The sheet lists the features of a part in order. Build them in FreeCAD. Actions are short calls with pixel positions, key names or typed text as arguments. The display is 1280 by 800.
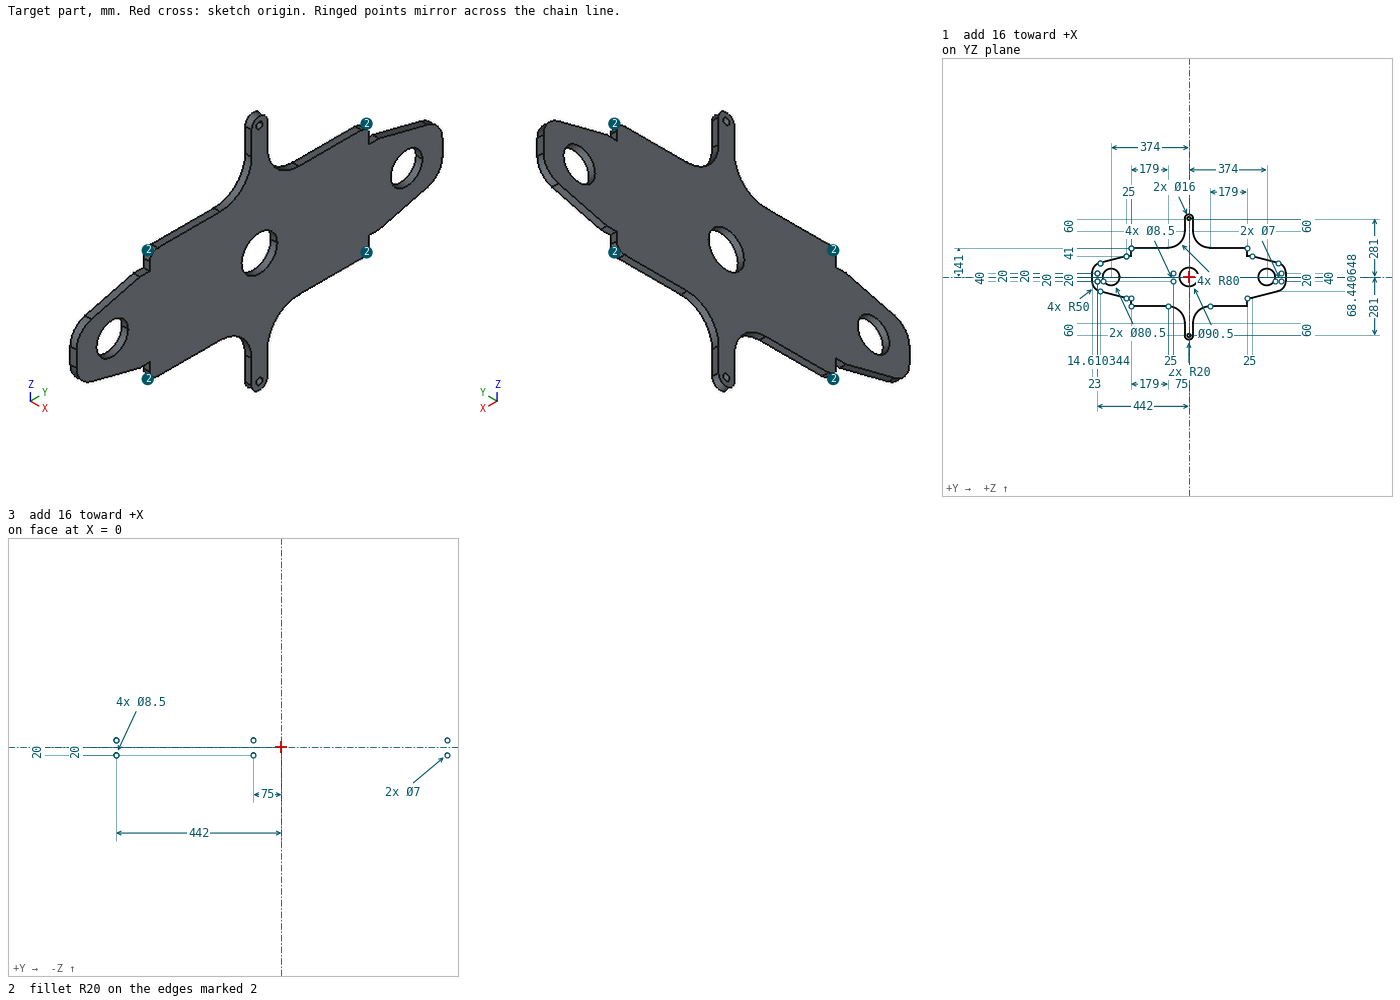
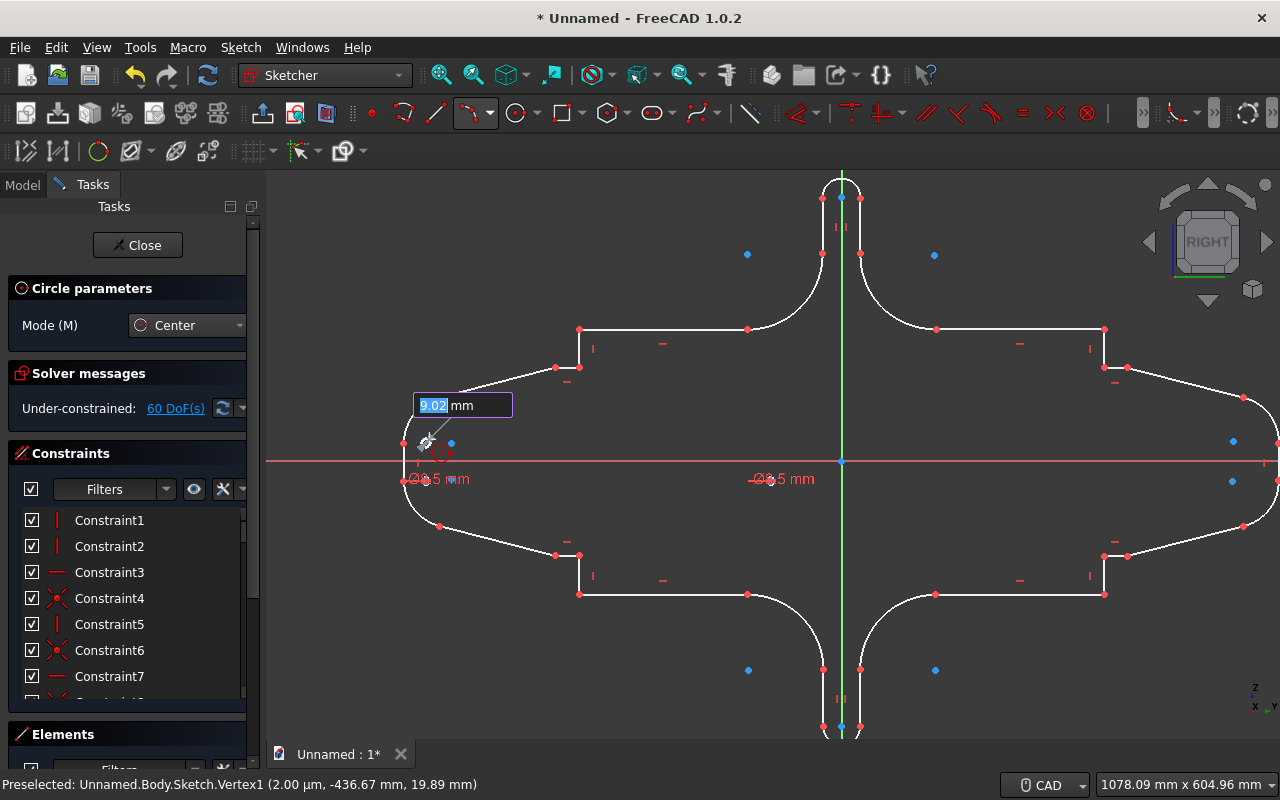
text(8.5)
key(Return)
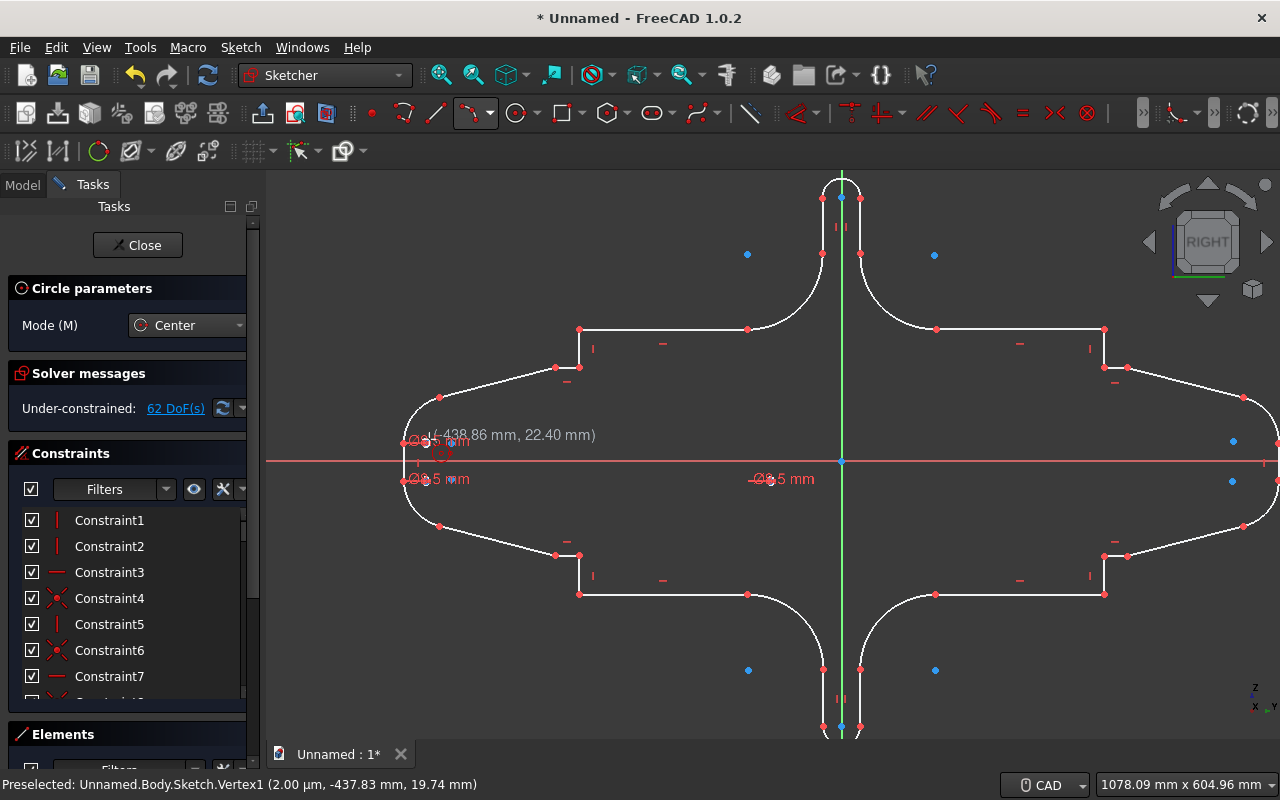
click(490, 461)
move(517, 434)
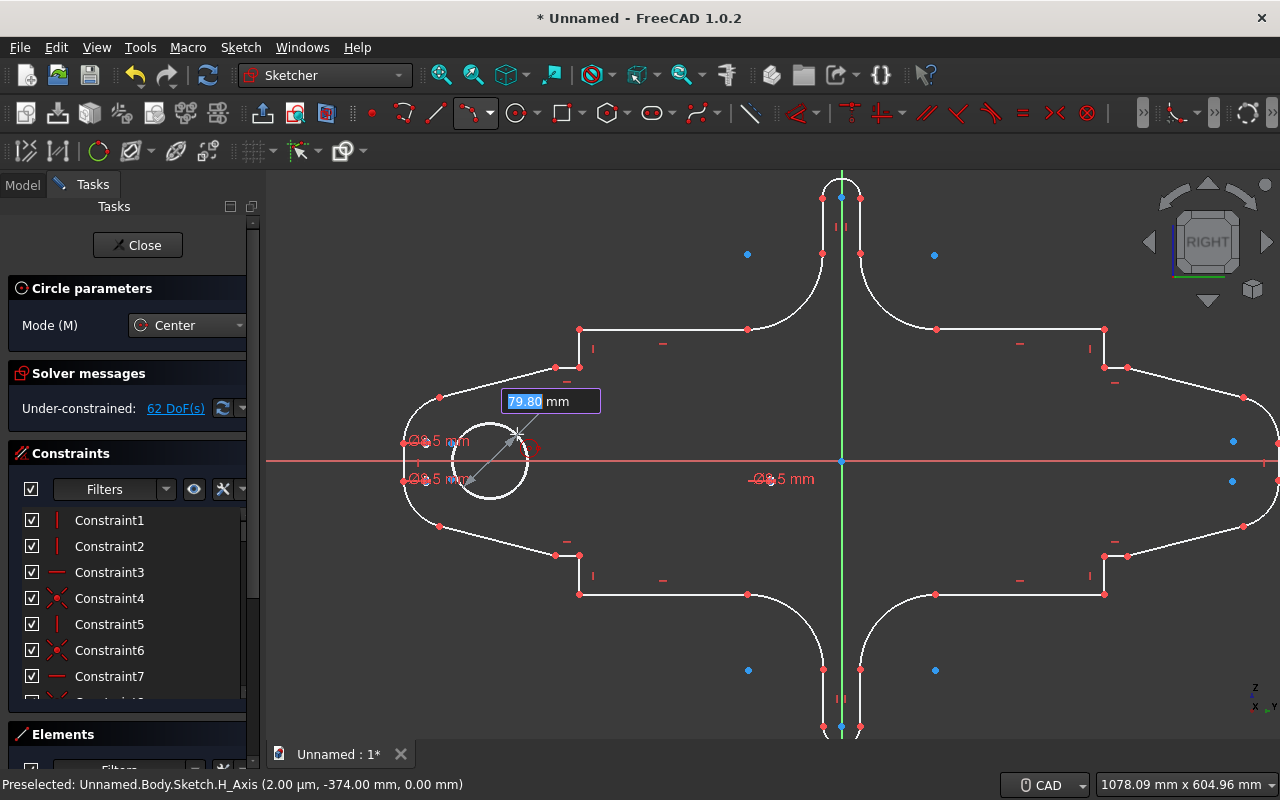
text(80.5)
key(Return)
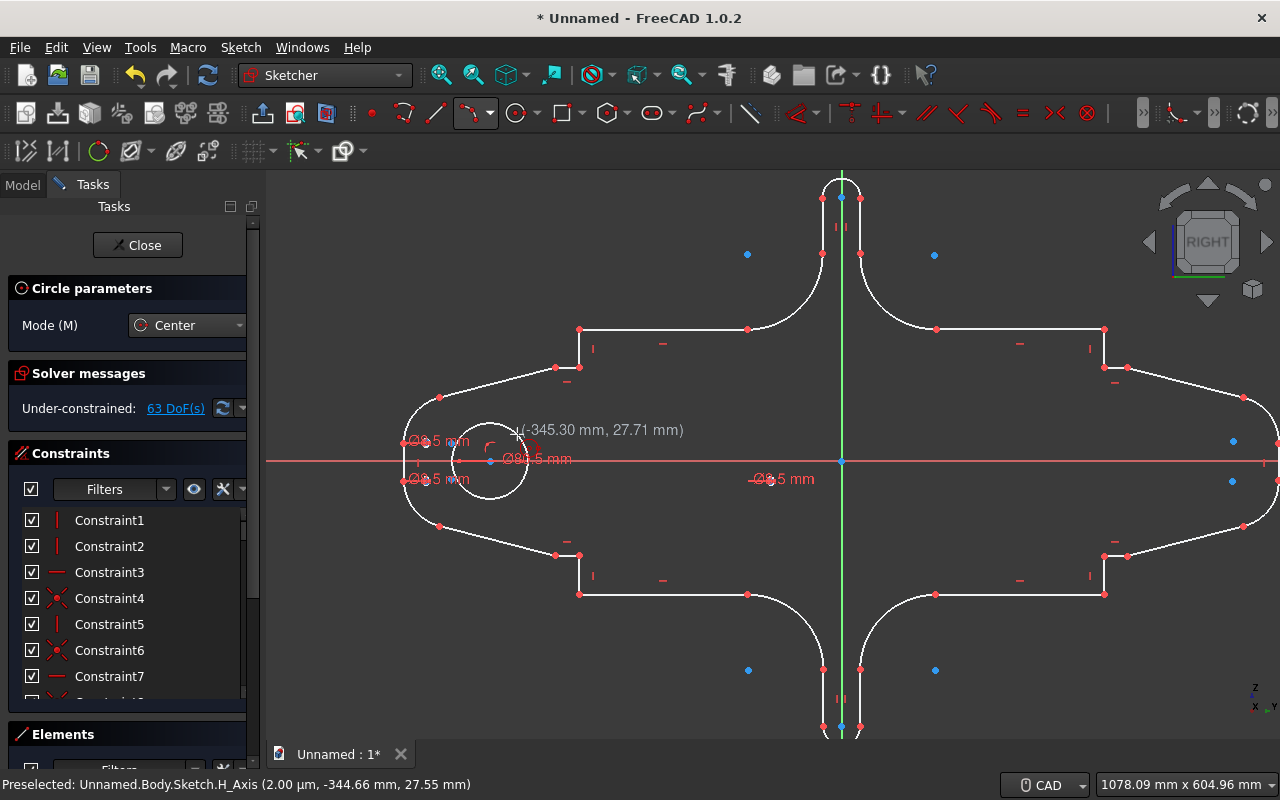
scroll(771, 442, up, 9)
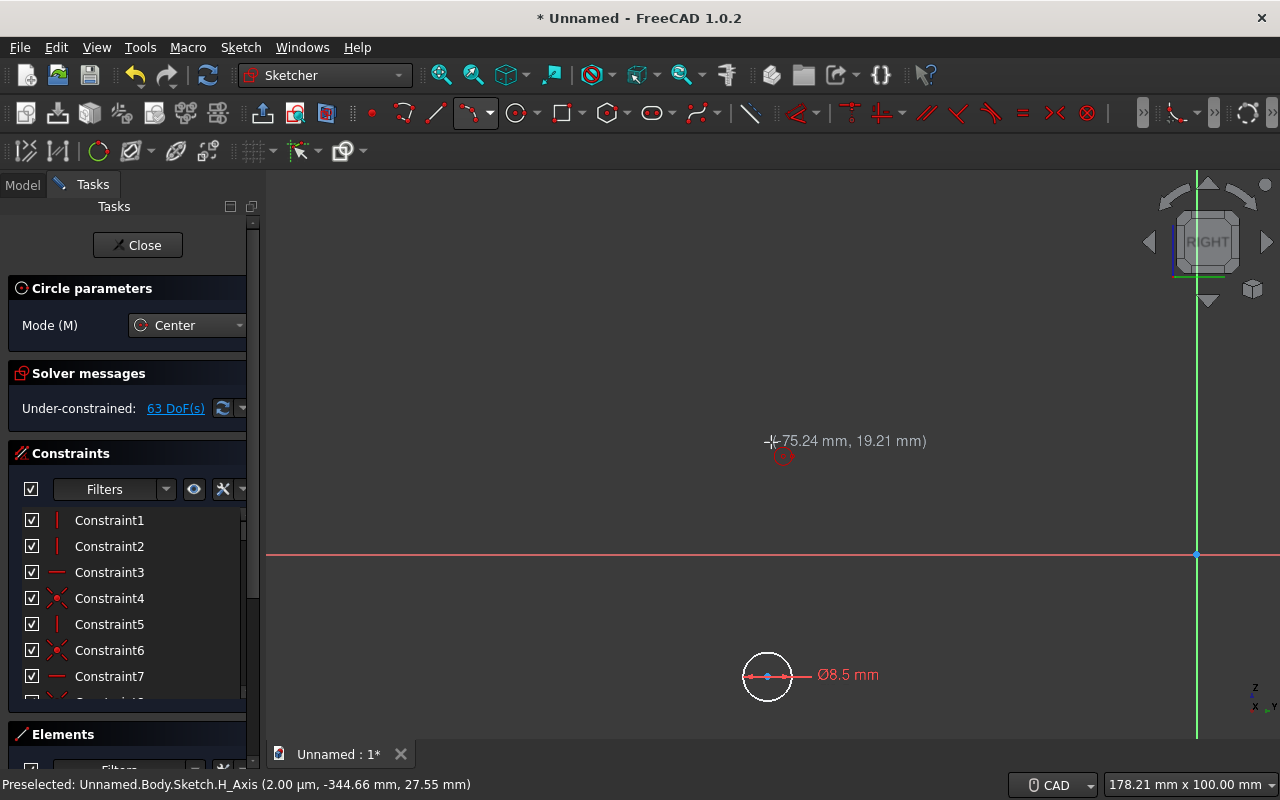
scroll(643, 442, down, 11)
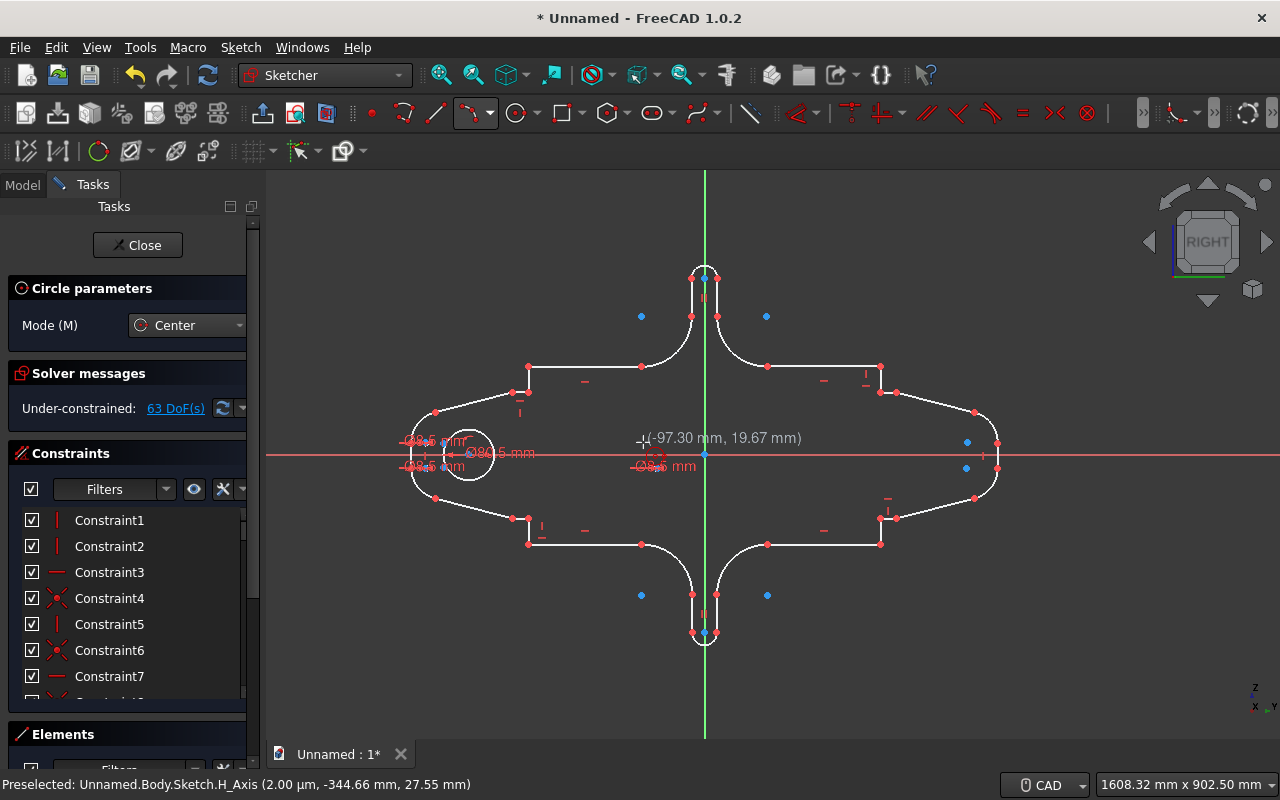
scroll(657, 442, up, 2)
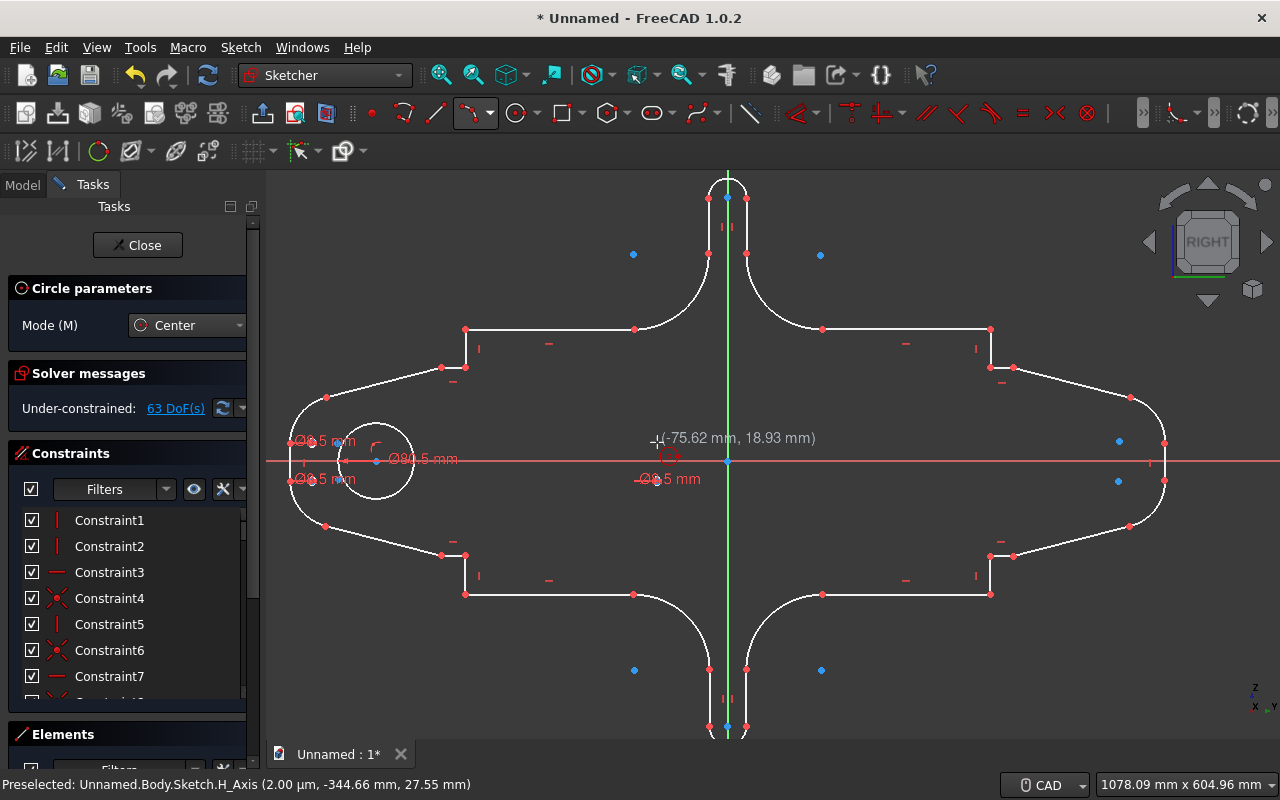
click(657, 442)
move(660, 439)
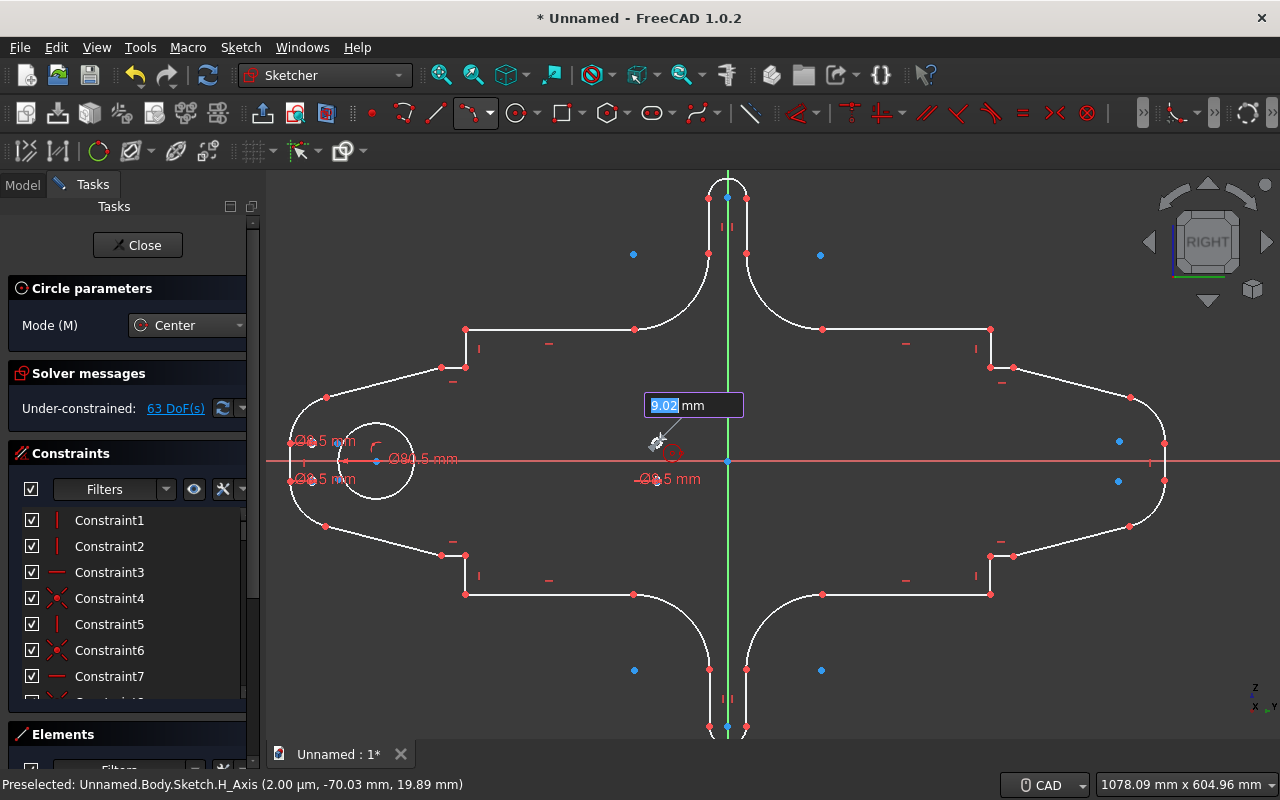
text(8.5)
key(Return)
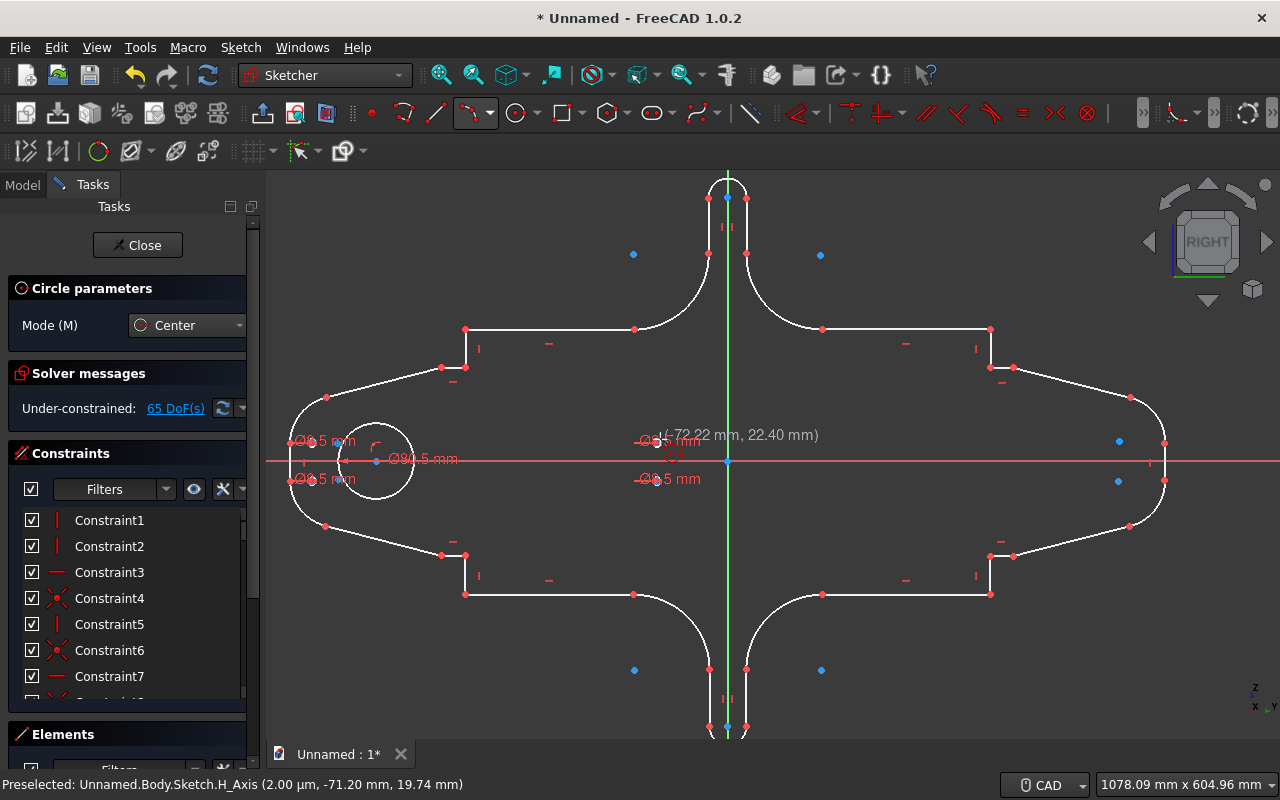
scroll(657, 441, down, 2)